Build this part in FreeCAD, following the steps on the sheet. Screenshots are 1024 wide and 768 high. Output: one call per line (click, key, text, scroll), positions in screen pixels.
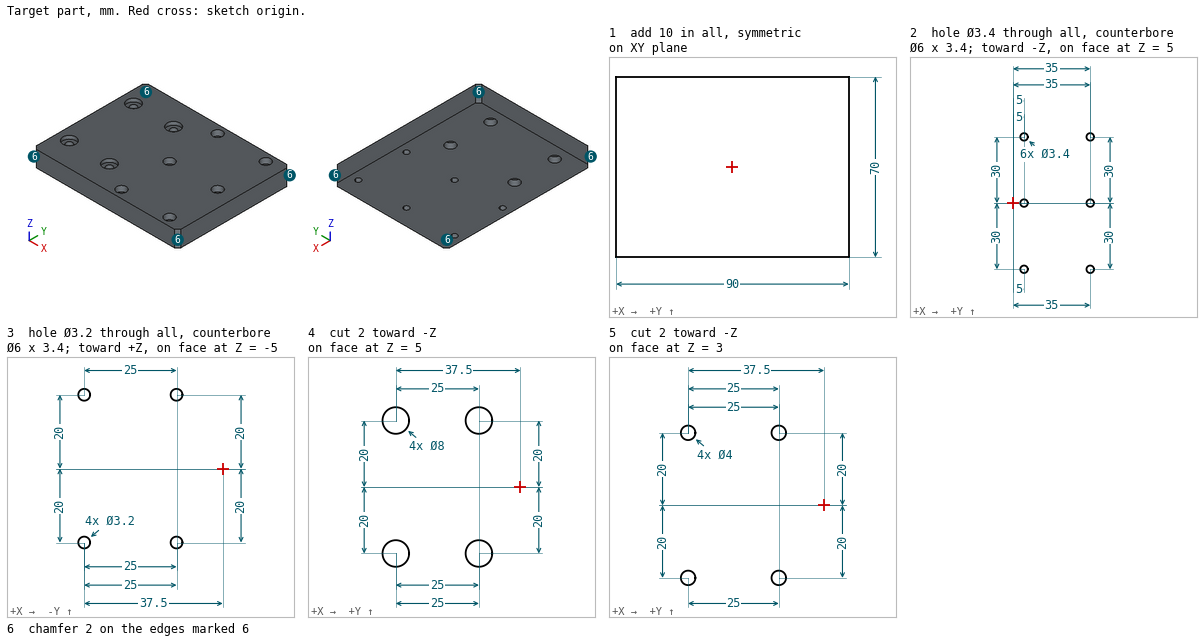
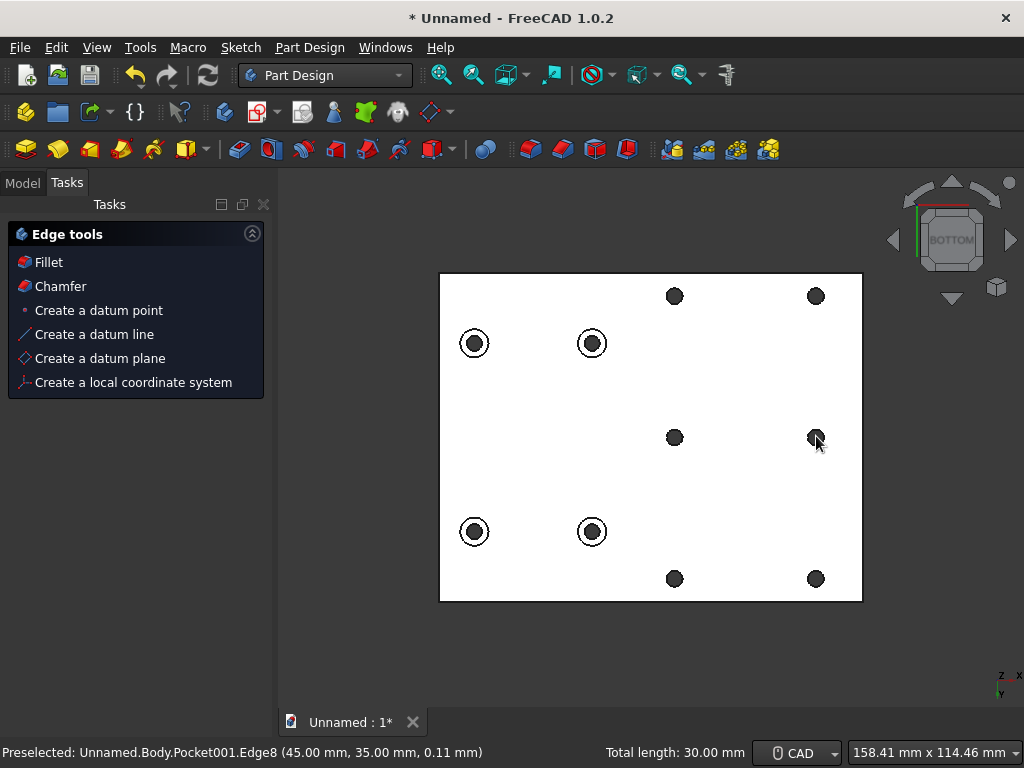
key(4)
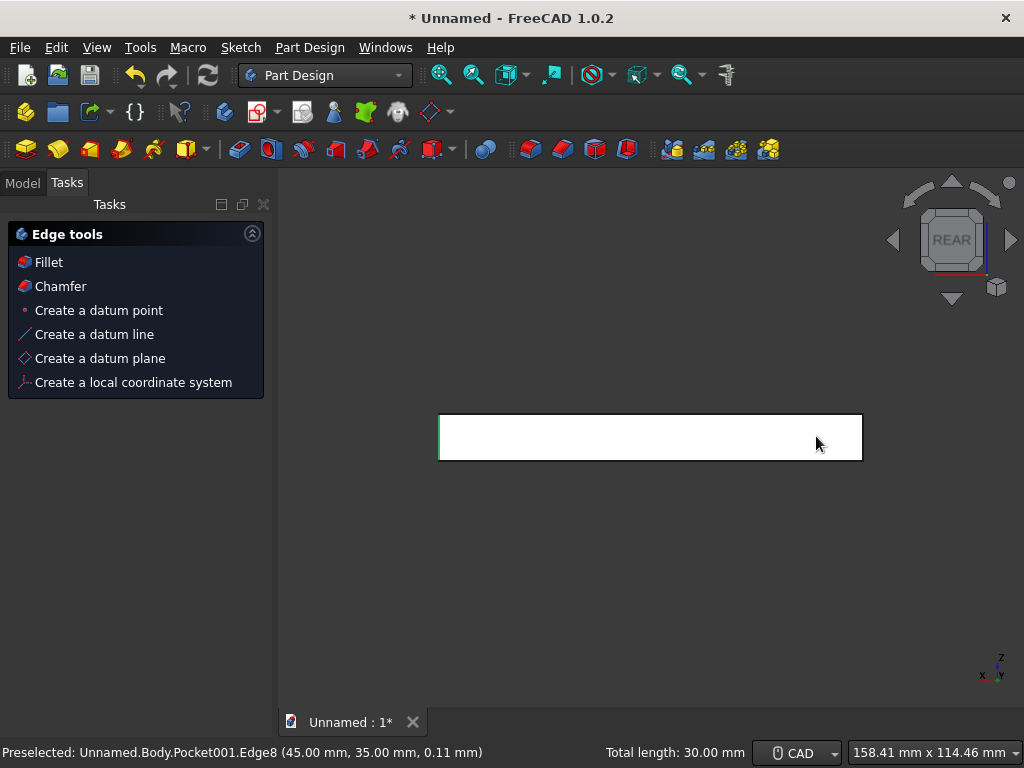
click(863, 437, ctrl)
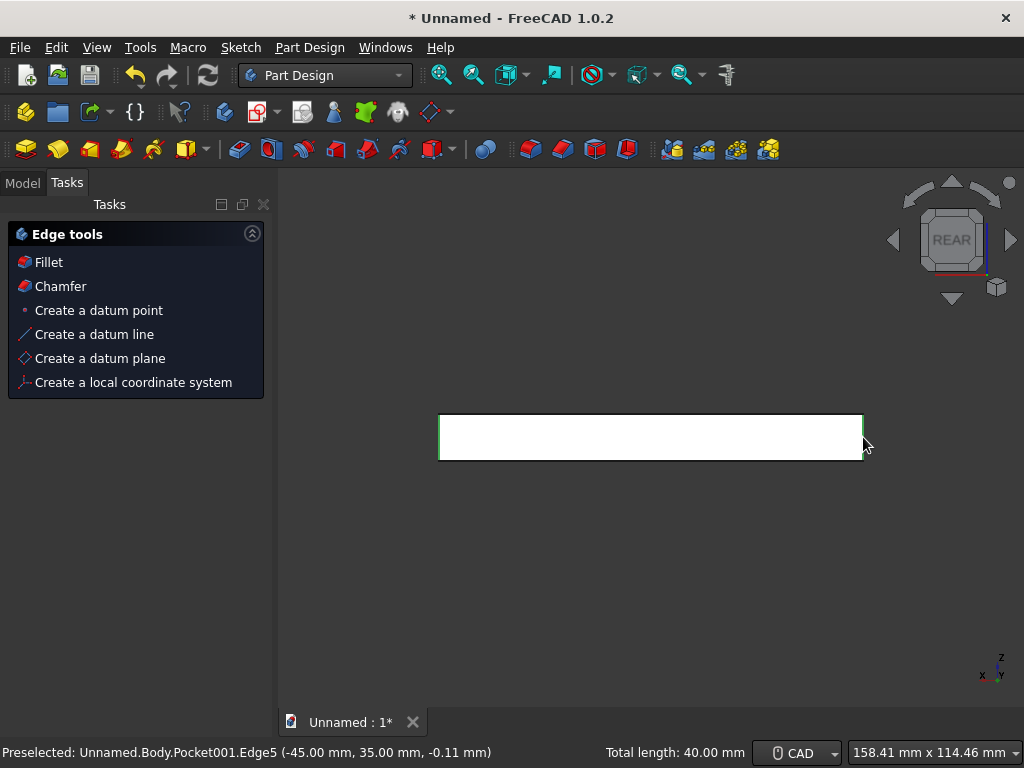
click(564, 150)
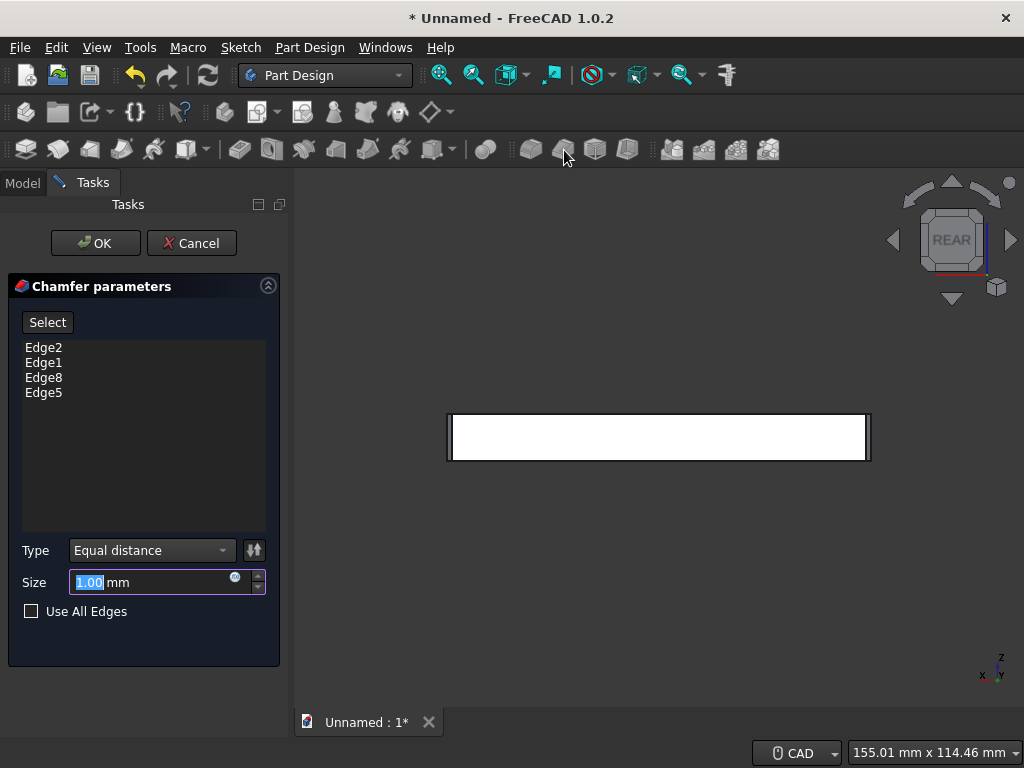
text(2)
key(Tab)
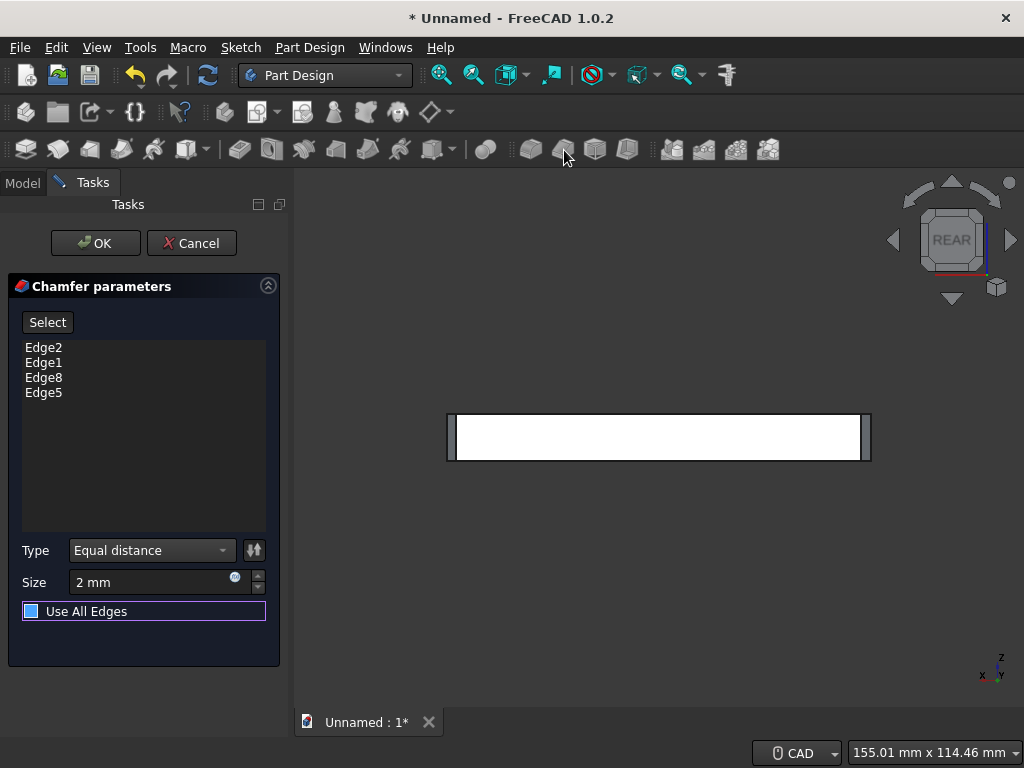
click(96, 243)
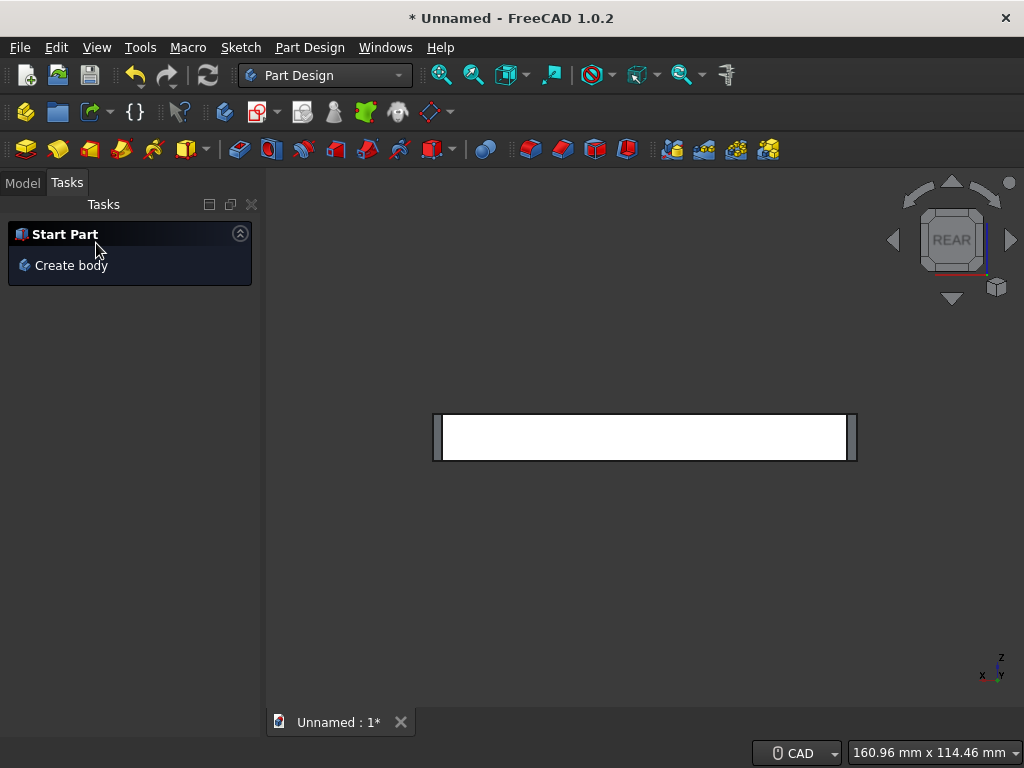
key(0)